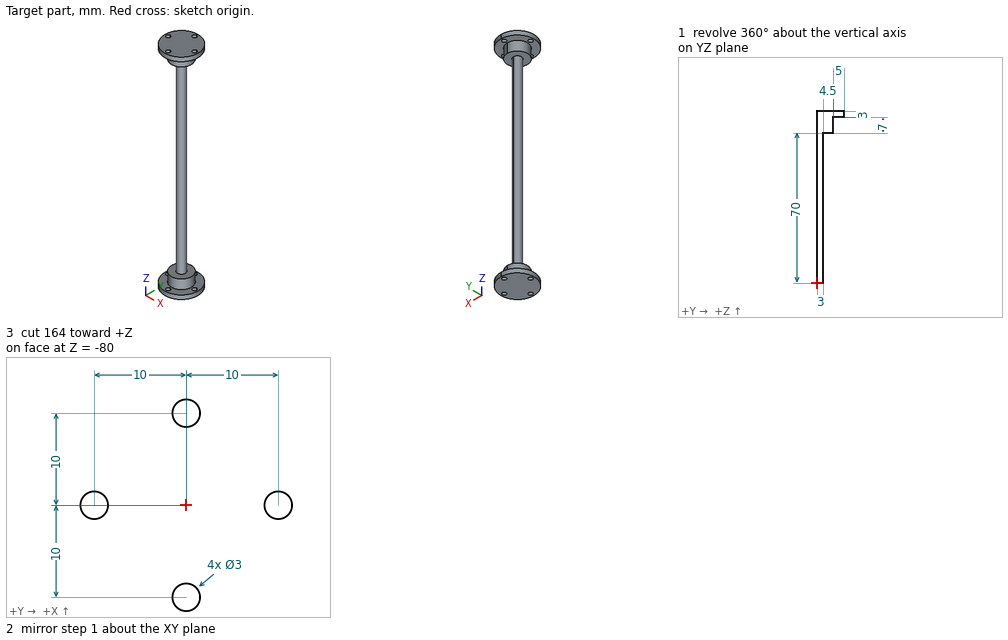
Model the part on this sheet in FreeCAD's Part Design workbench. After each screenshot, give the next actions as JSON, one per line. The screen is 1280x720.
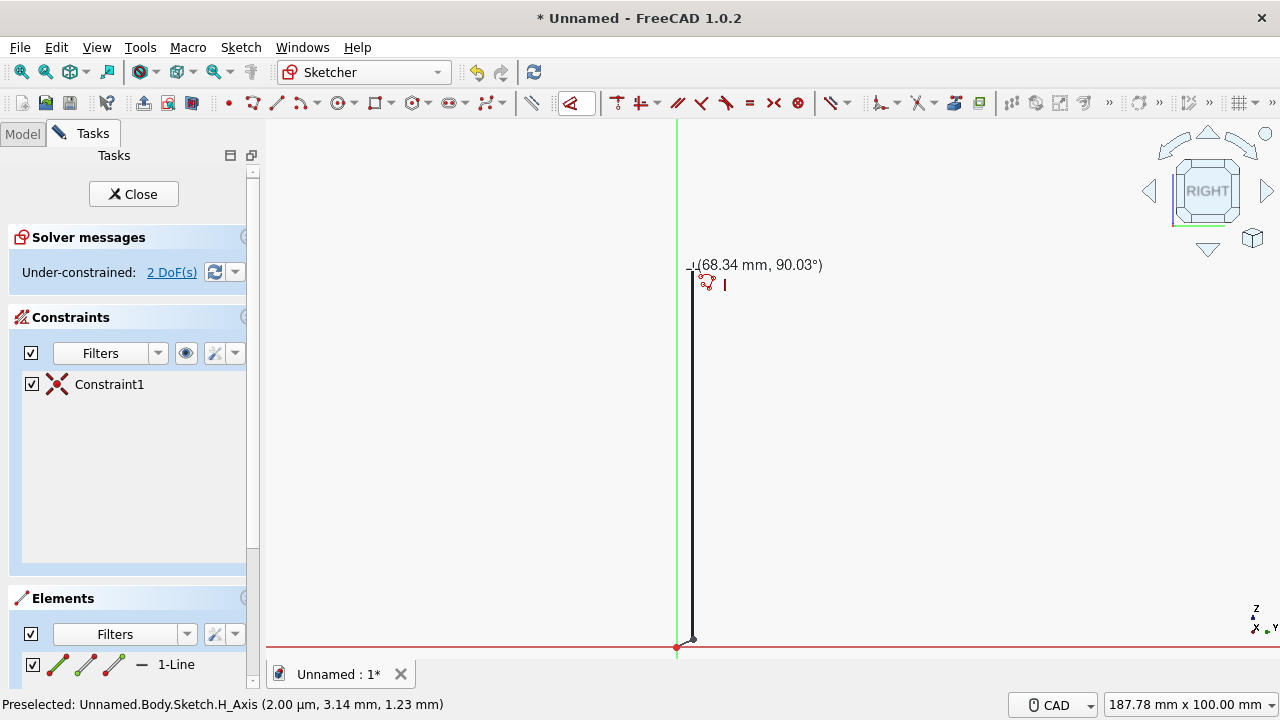
{"action": "left_click", "coordinate": [693, 269]}
{"action": "left_click", "coordinate": [717, 269]}
{"action": "left_click", "coordinate": [717, 231]}
{"action": "left_click", "coordinate": [744, 231]}
{"action": "left_click", "coordinate": [744, 215]}
{"action": "left_click", "coordinate": [686, 215]}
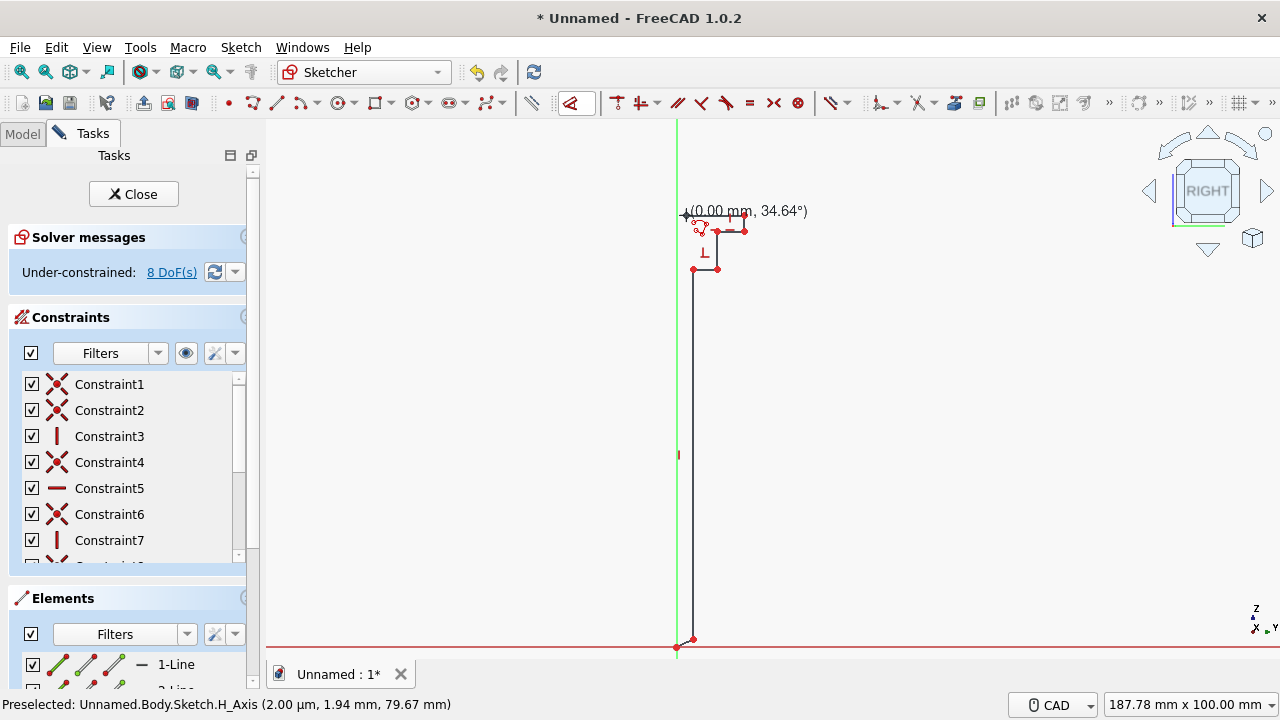
{"action": "scroll", "coordinate": [678, 198], "scroll_direction": "down", "scroll_amount": 1}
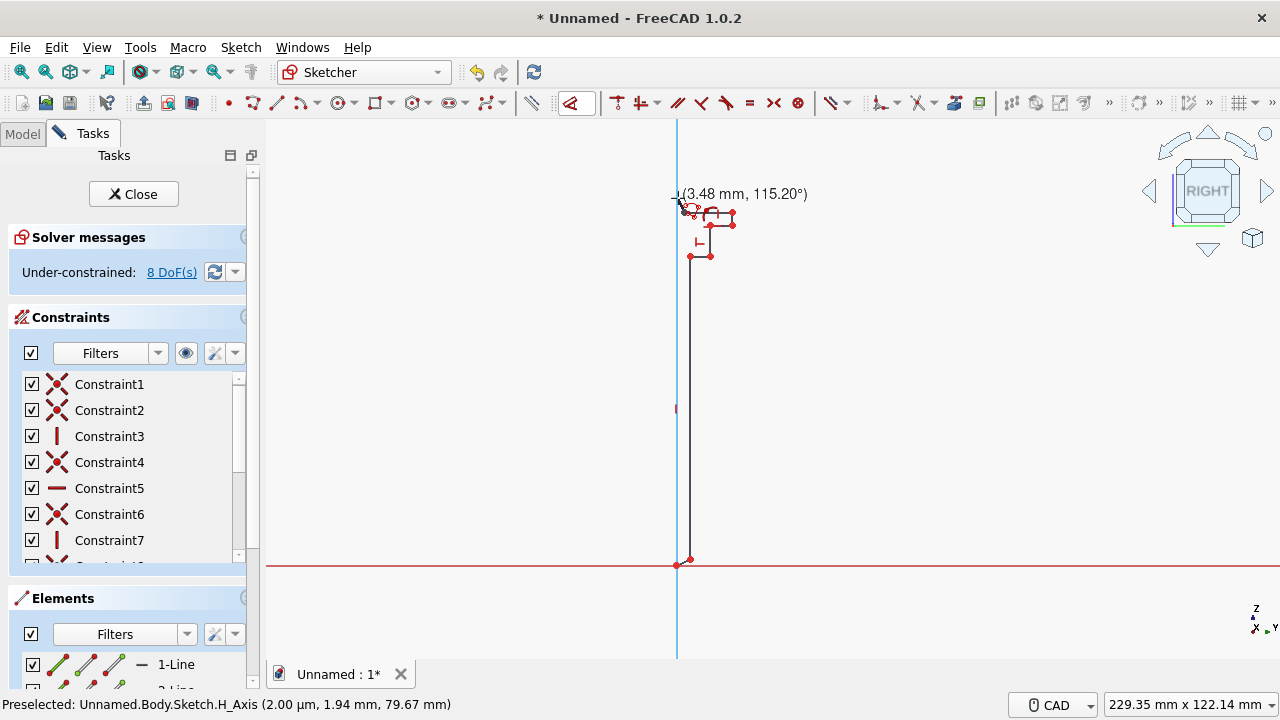
{"action": "scroll", "coordinate": [677, 566], "scroll_direction": "up", "scroll_amount": 5}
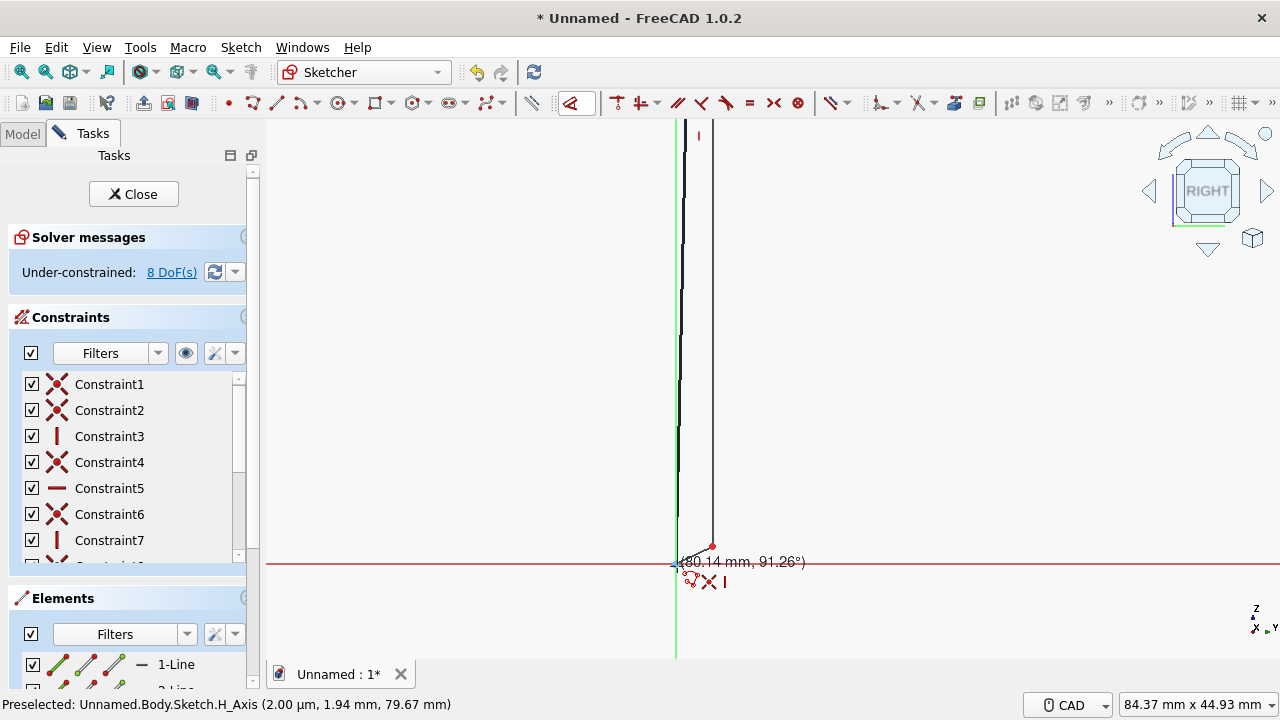
{"action": "left_click", "coordinate": [676, 564]}
{"action": "key", "text": "Escape"}
{"action": "key", "text": "Escape"}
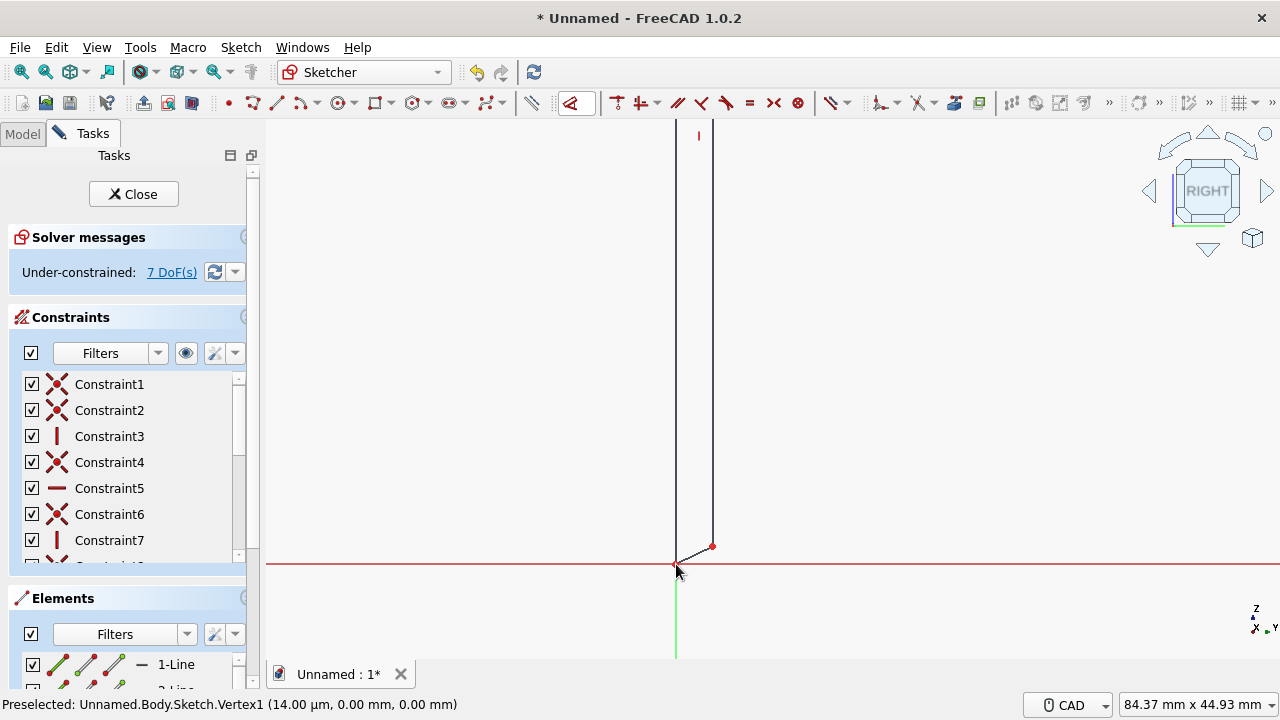
{"action": "left_click", "coordinate": [702, 552]}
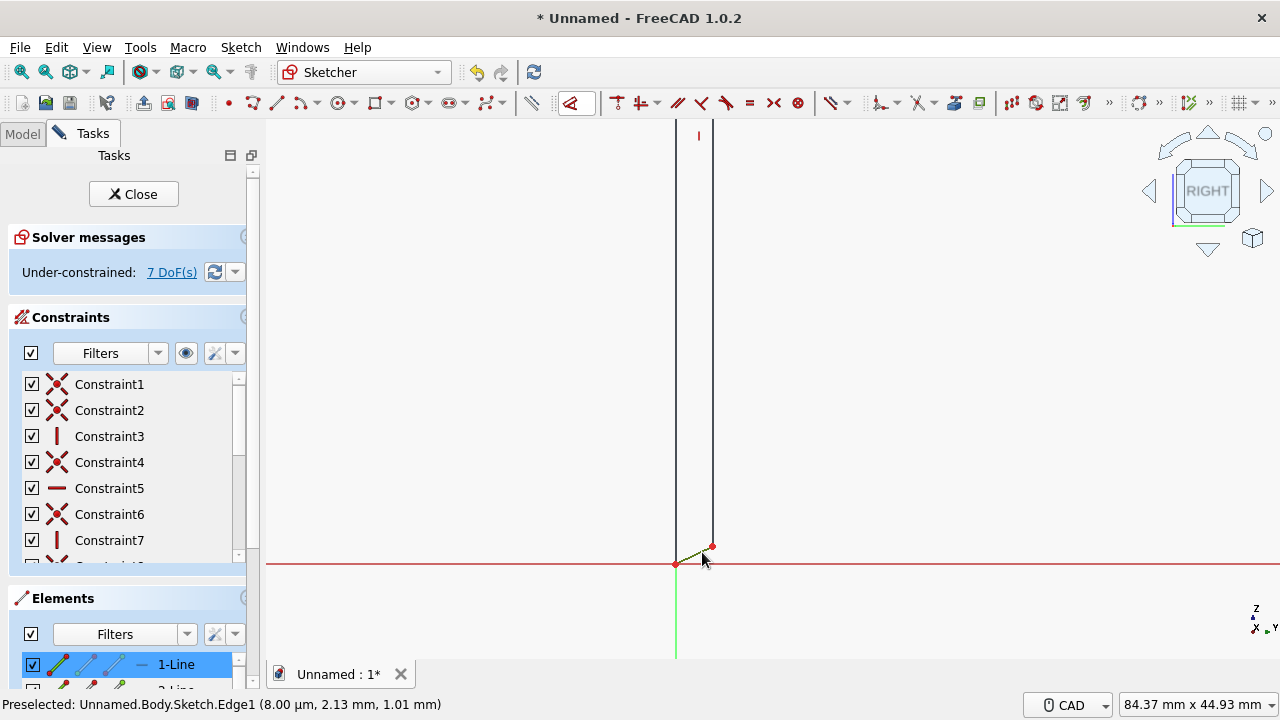
{"action": "left_click", "coordinate": [660, 104]}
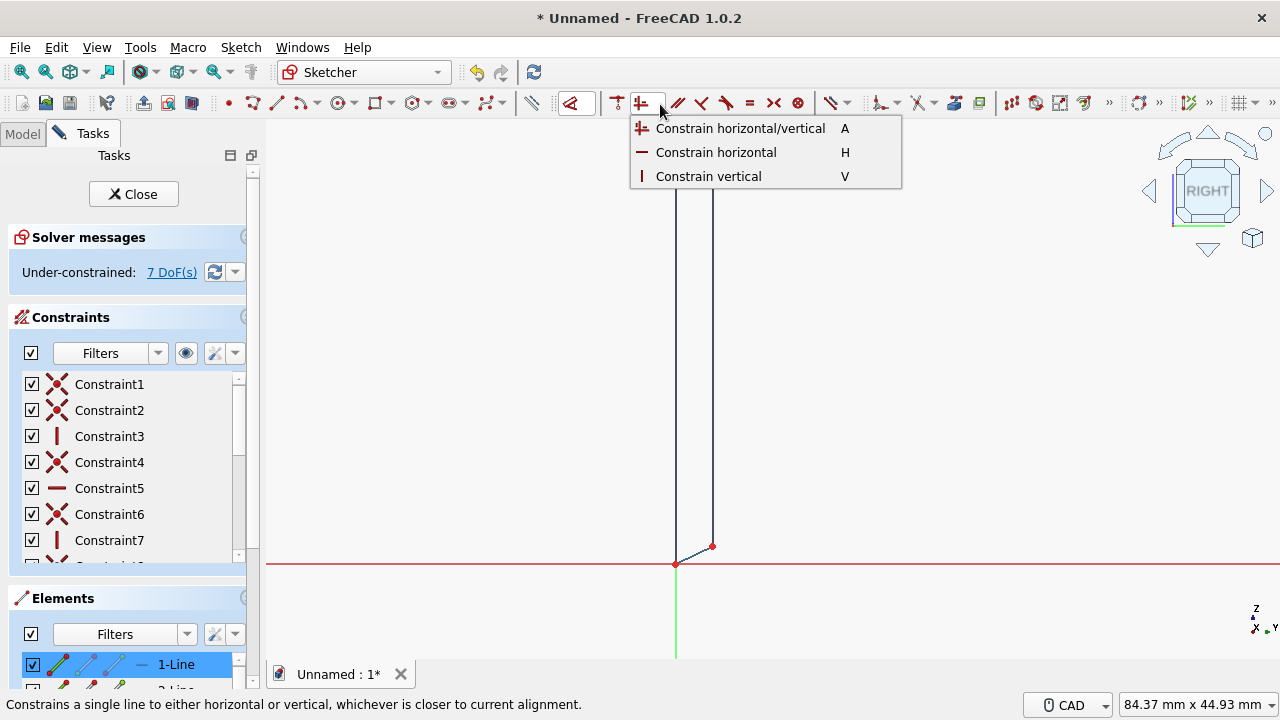
{"action": "left_click", "coordinate": [766, 152]}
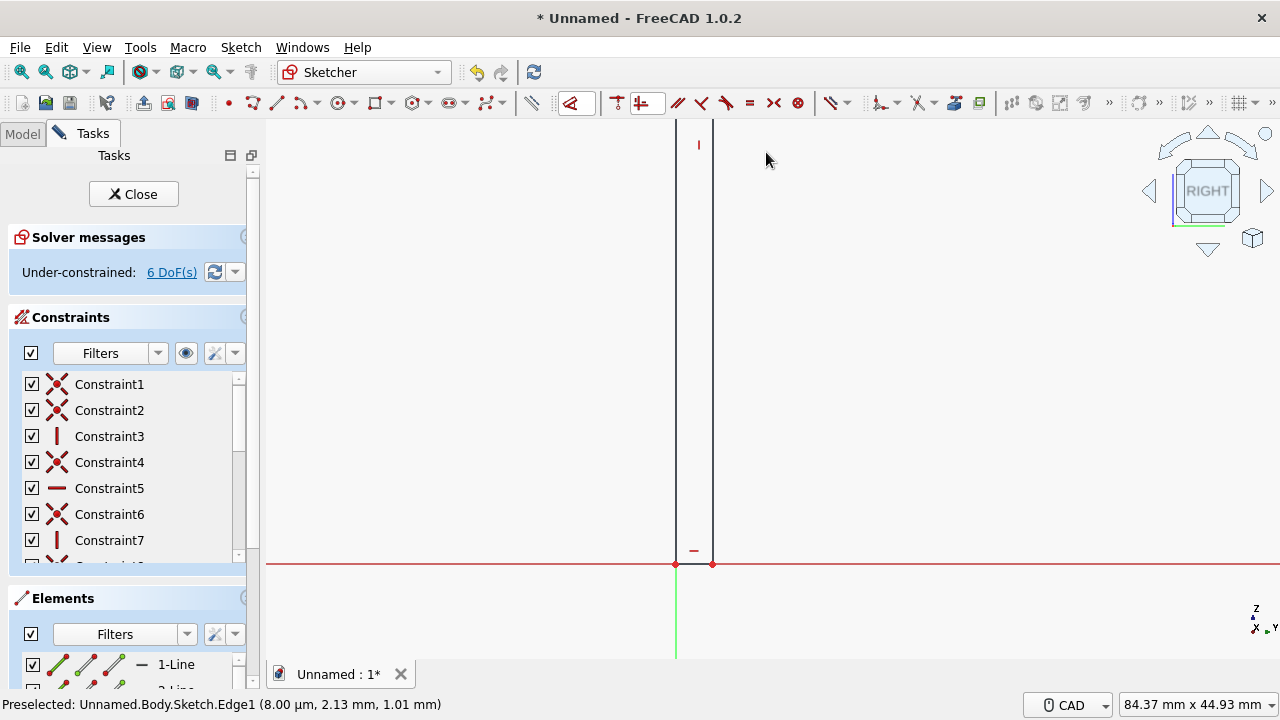
{"action": "left_click", "coordinate": [570, 104]}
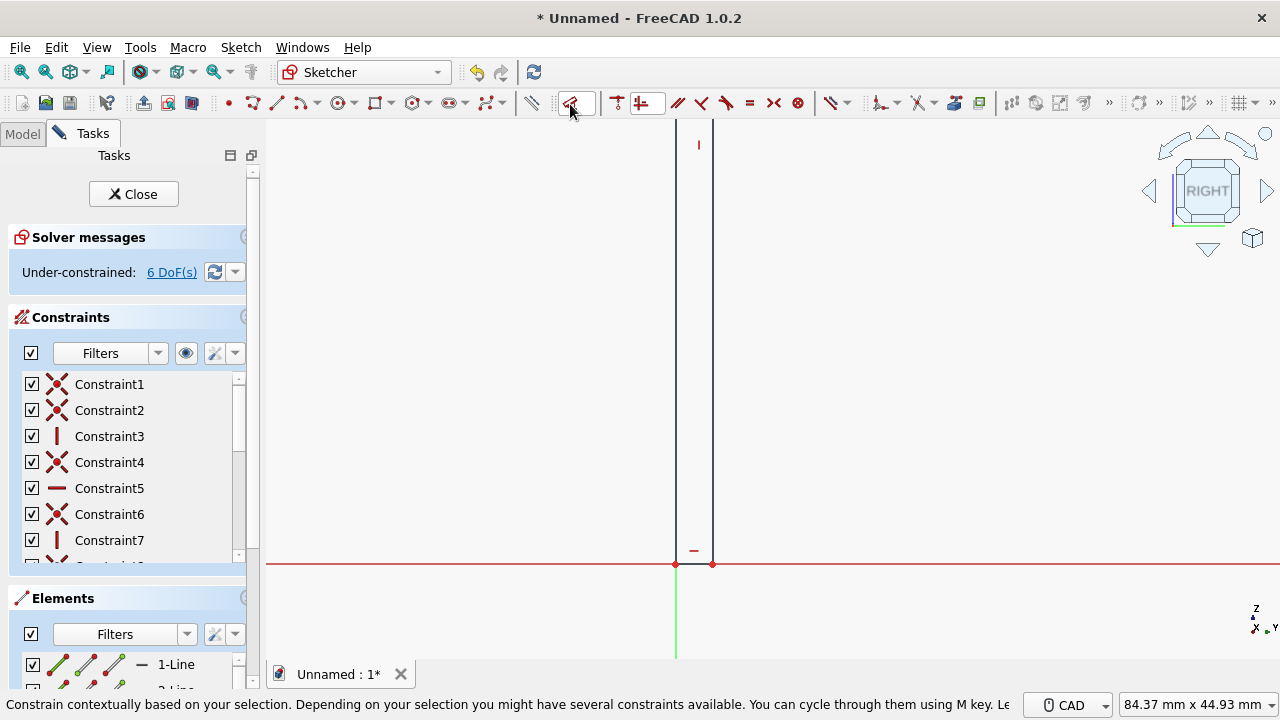
{"action": "scroll", "coordinate": [687, 564], "scroll_direction": "up", "scroll_amount": 2}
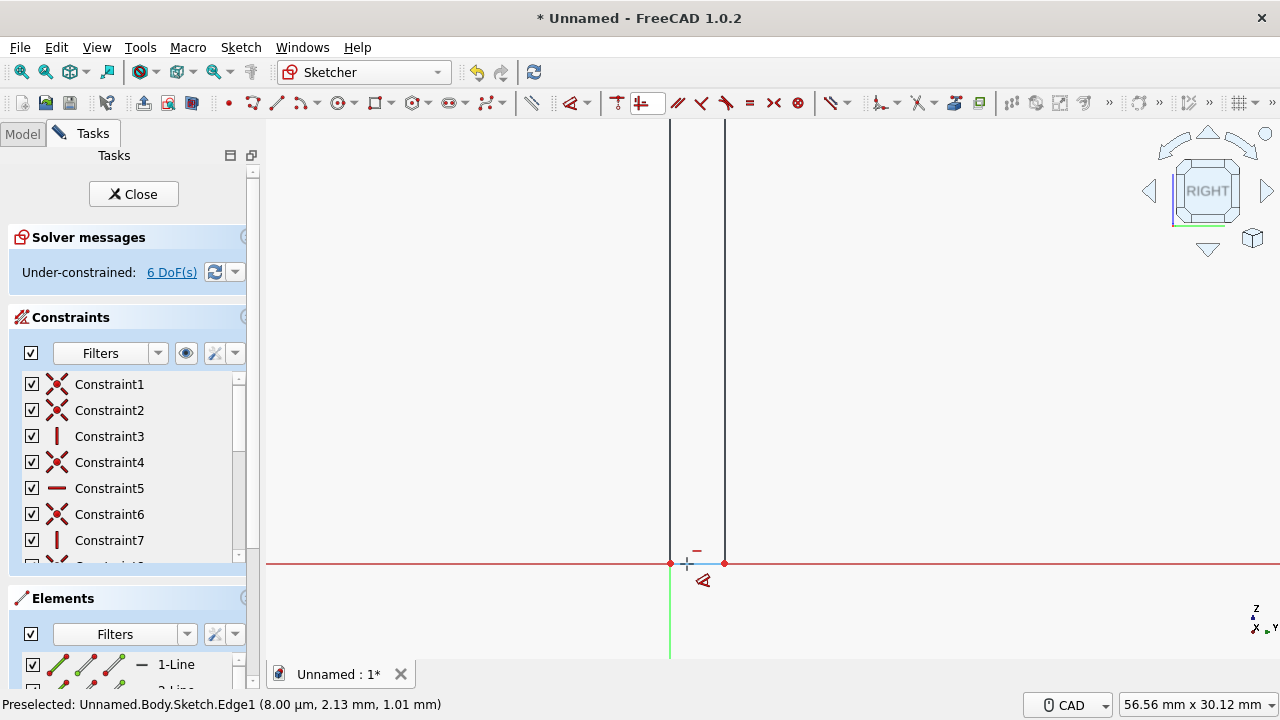
{"action": "left_click", "coordinate": [687, 564]}
{"action": "left_click", "coordinate": [698, 598]}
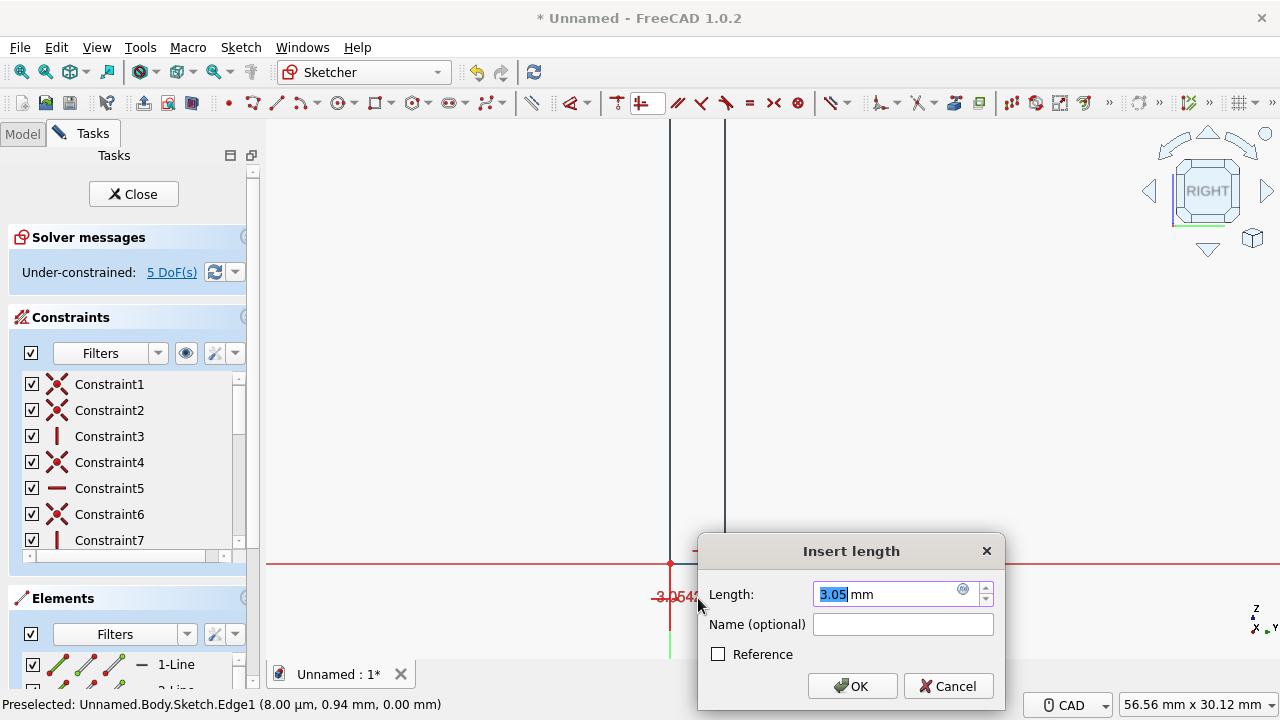
{"action": "type", "text": "3"}
{"action": "key", "text": "Return"}